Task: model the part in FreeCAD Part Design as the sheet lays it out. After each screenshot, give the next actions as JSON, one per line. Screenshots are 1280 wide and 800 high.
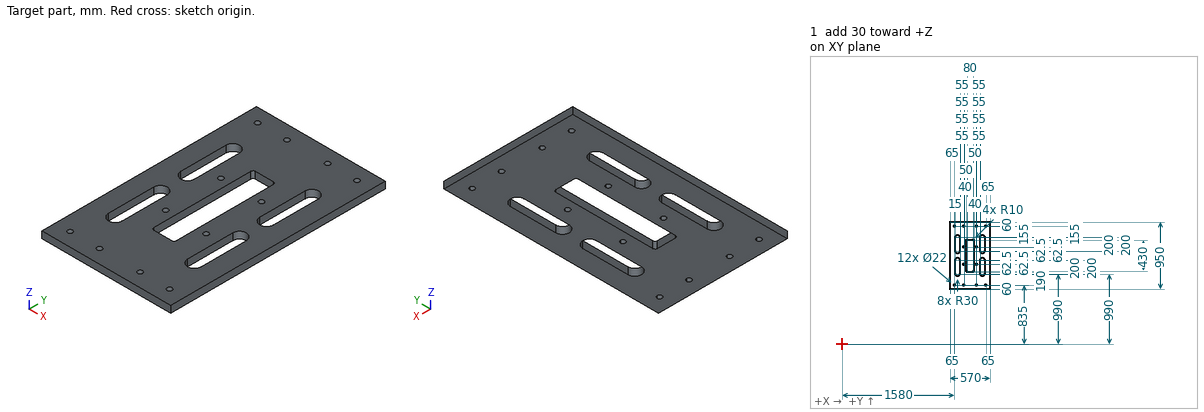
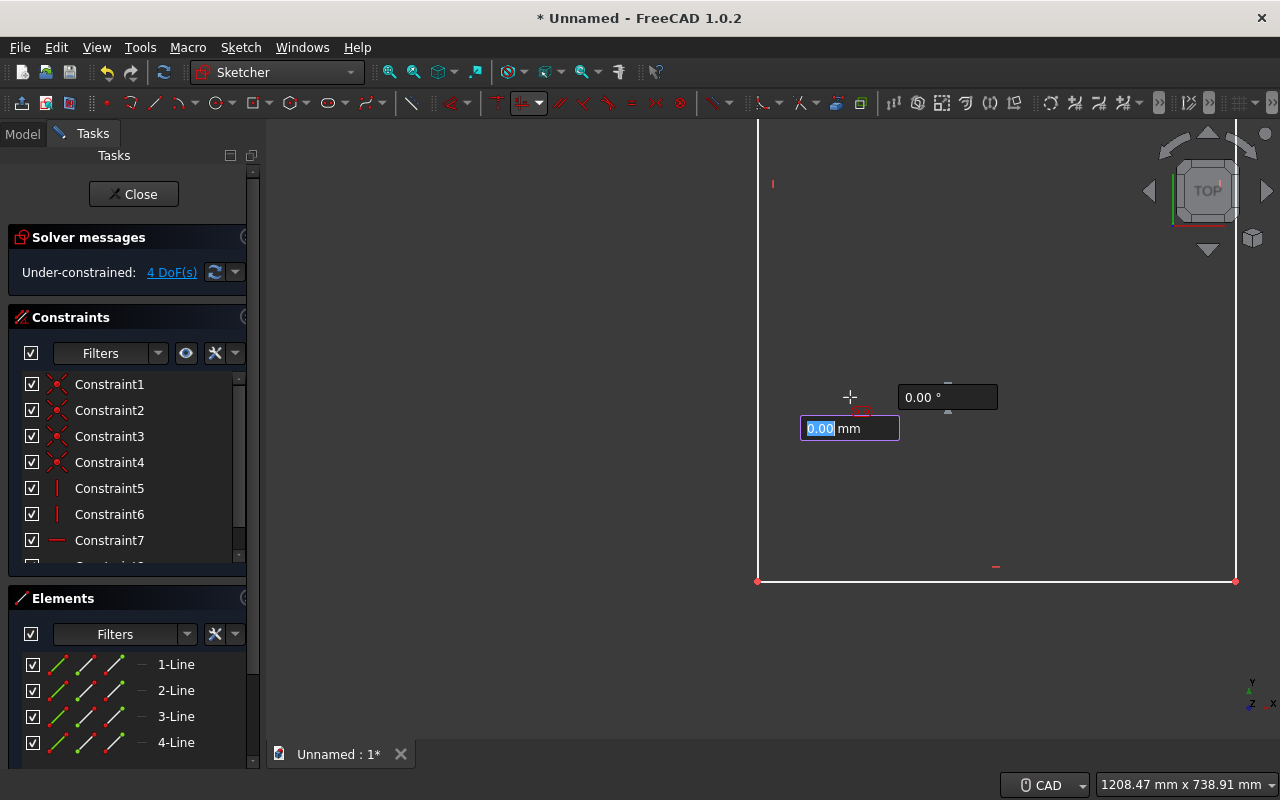
{"action": "left_click", "coordinate": [850, 229]}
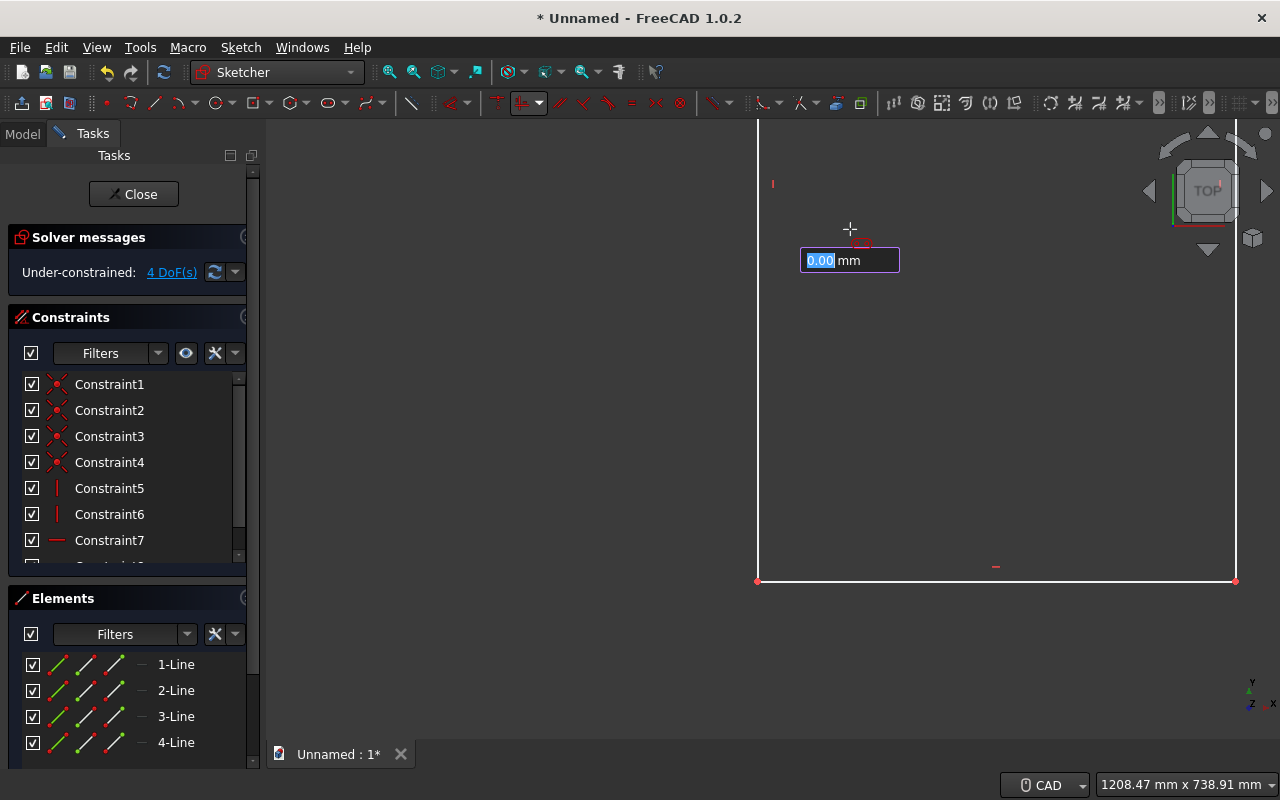
{"action": "left_click", "coordinate": [876, 313]}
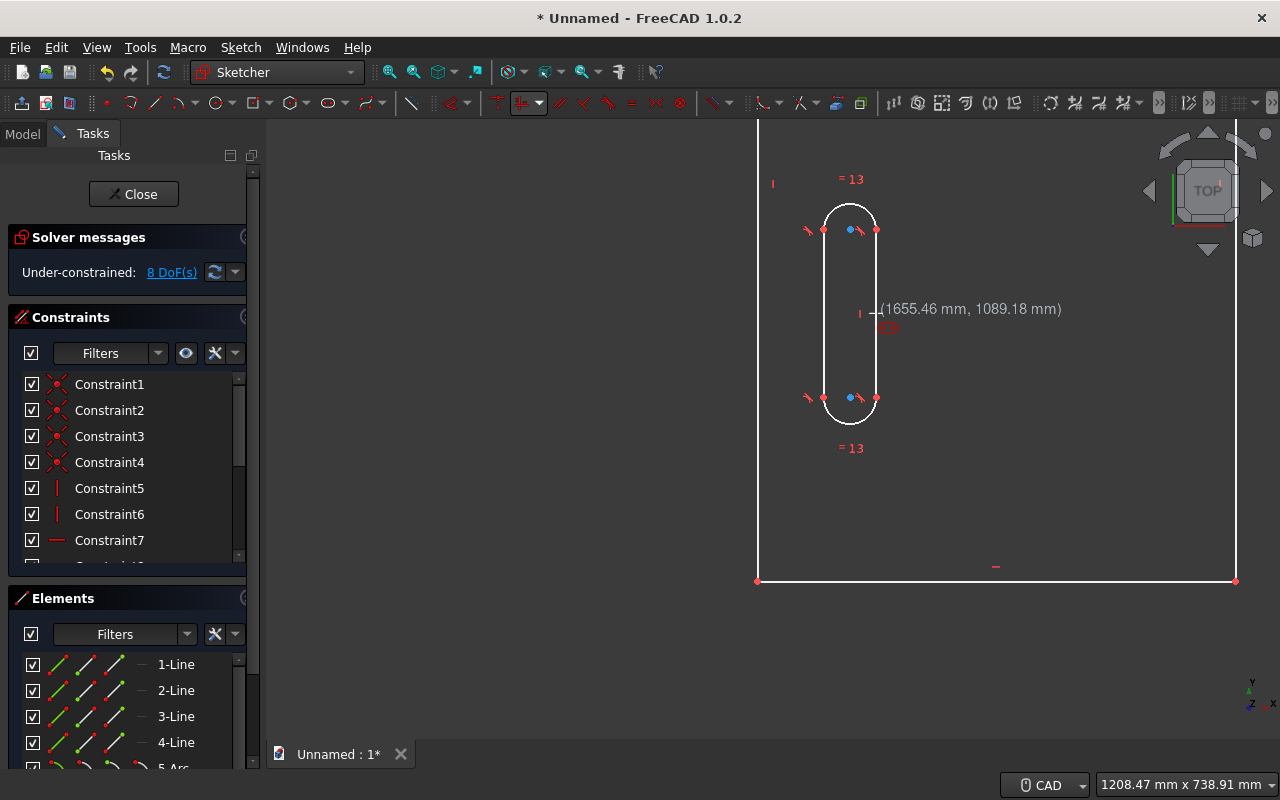
{"action": "scroll", "coordinate": [852, 397], "scroll_direction": "down", "scroll_amount": 6}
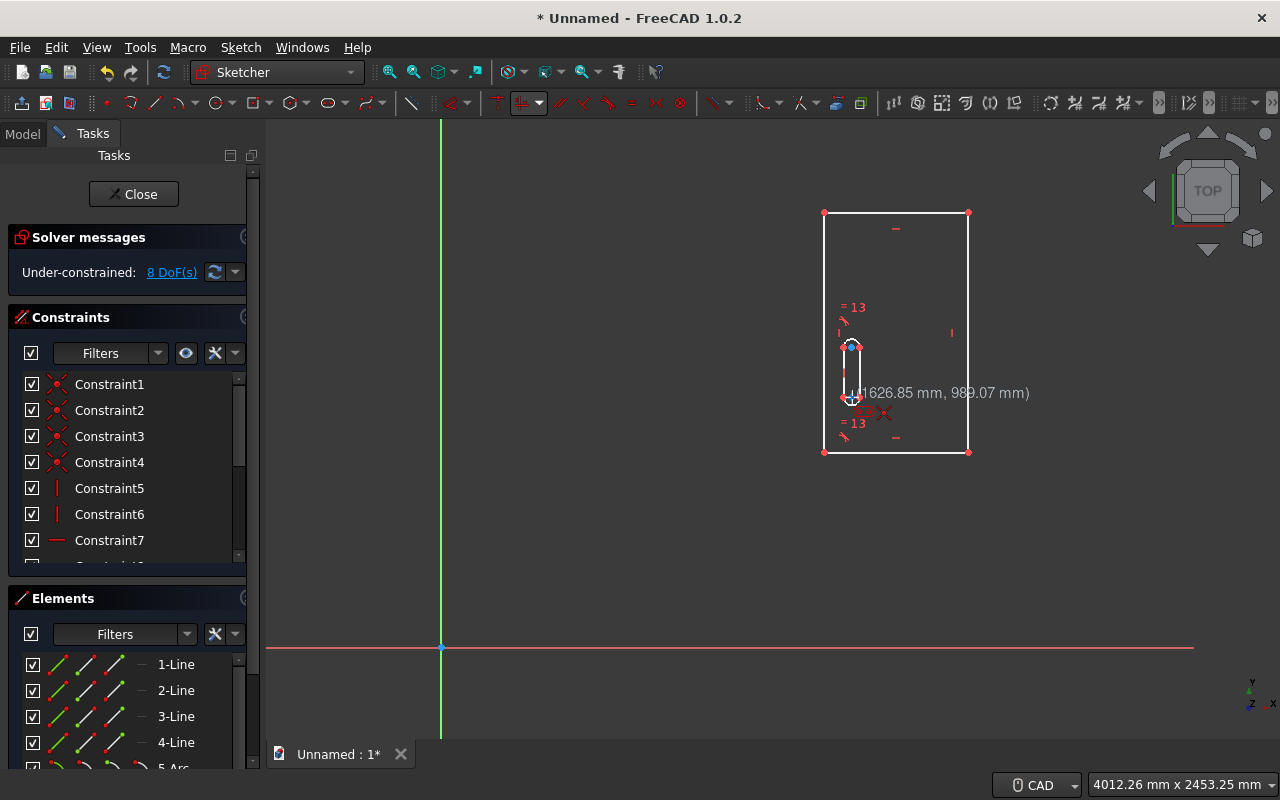
{"action": "scroll", "coordinate": [940, 397], "scroll_direction": "up", "scroll_amount": 6}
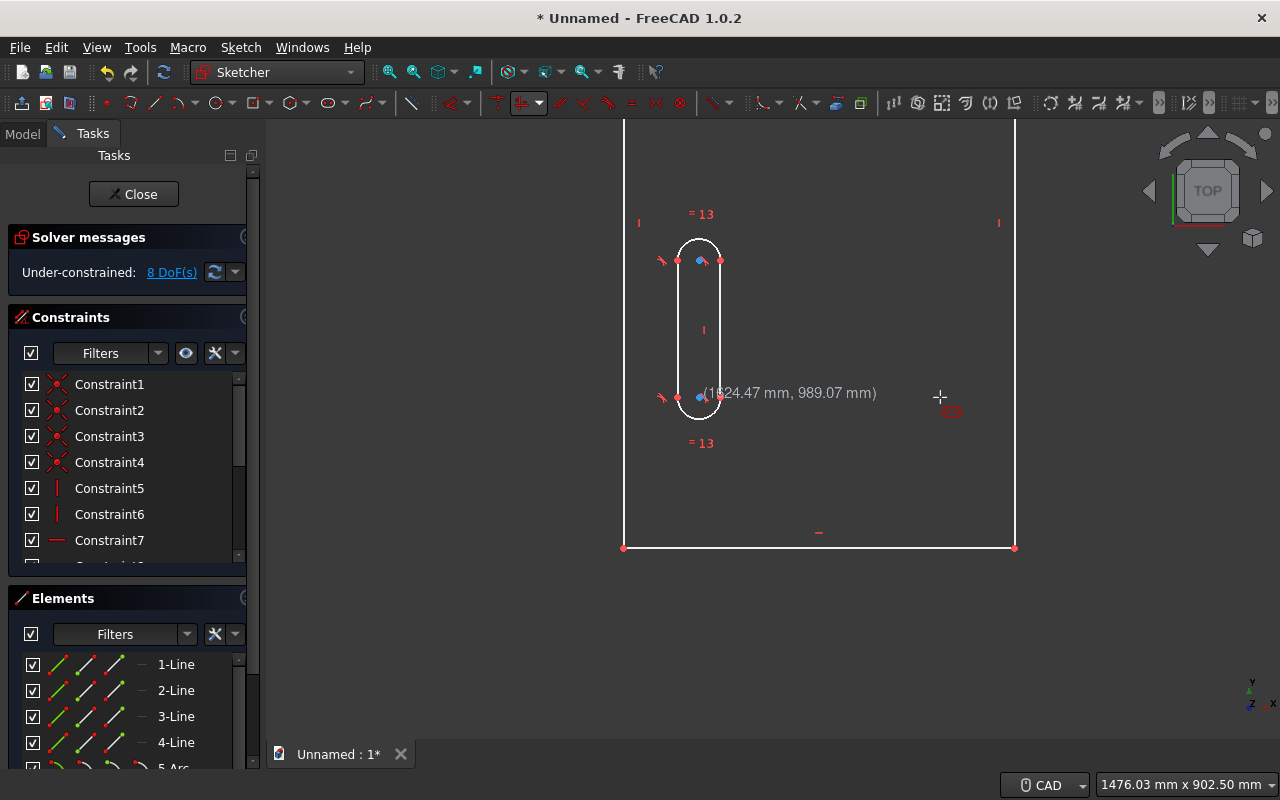
{"action": "left_click", "coordinate": [940, 397]}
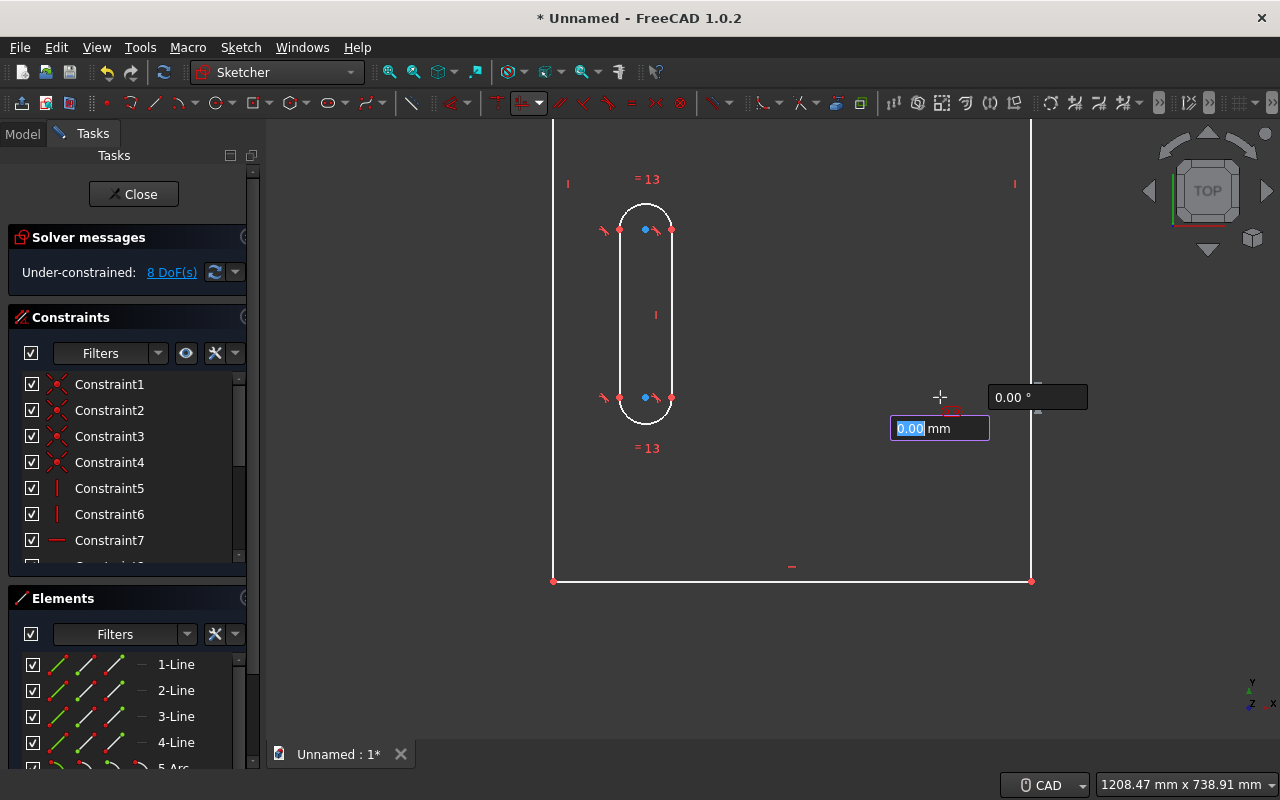
{"action": "left_click", "coordinate": [940, 229]}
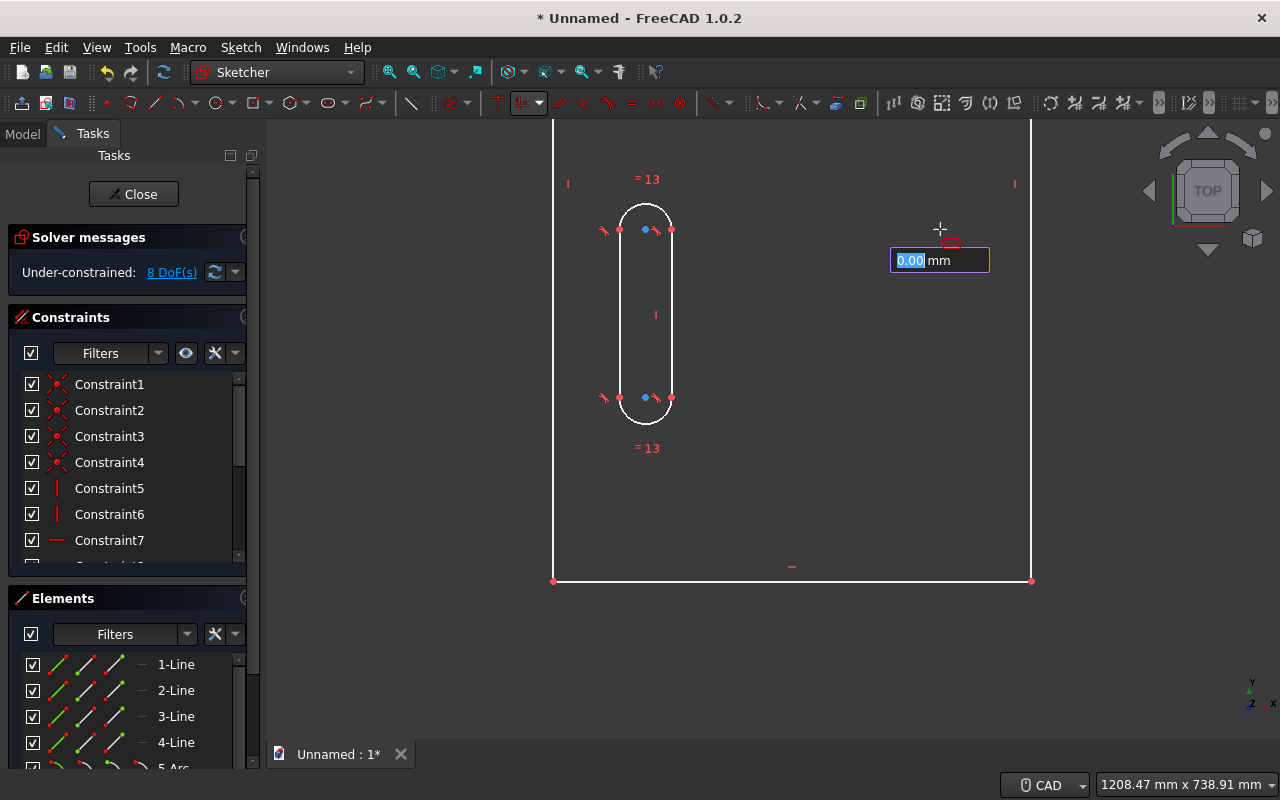
{"action": "left_click", "coordinate": [965, 313]}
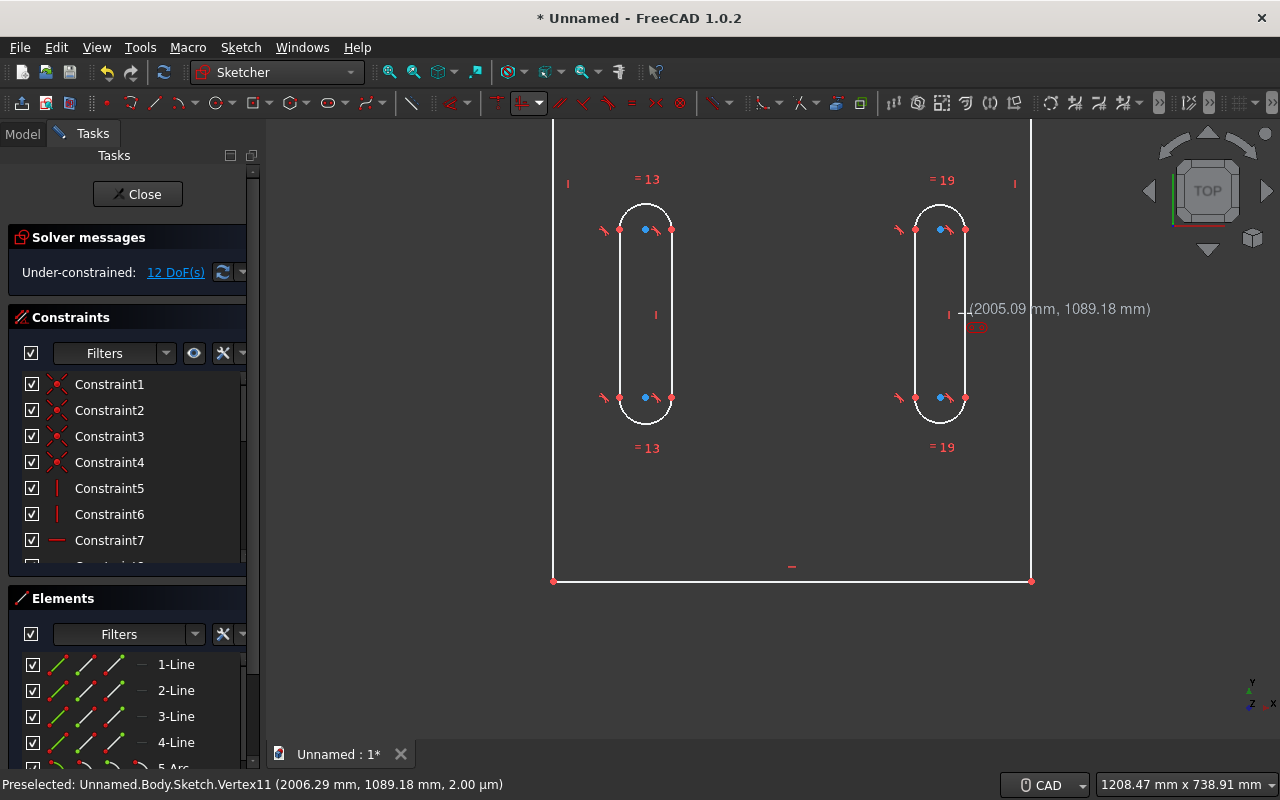
{"action": "scroll", "coordinate": [940, 397], "scroll_direction": "down", "scroll_amount": 6}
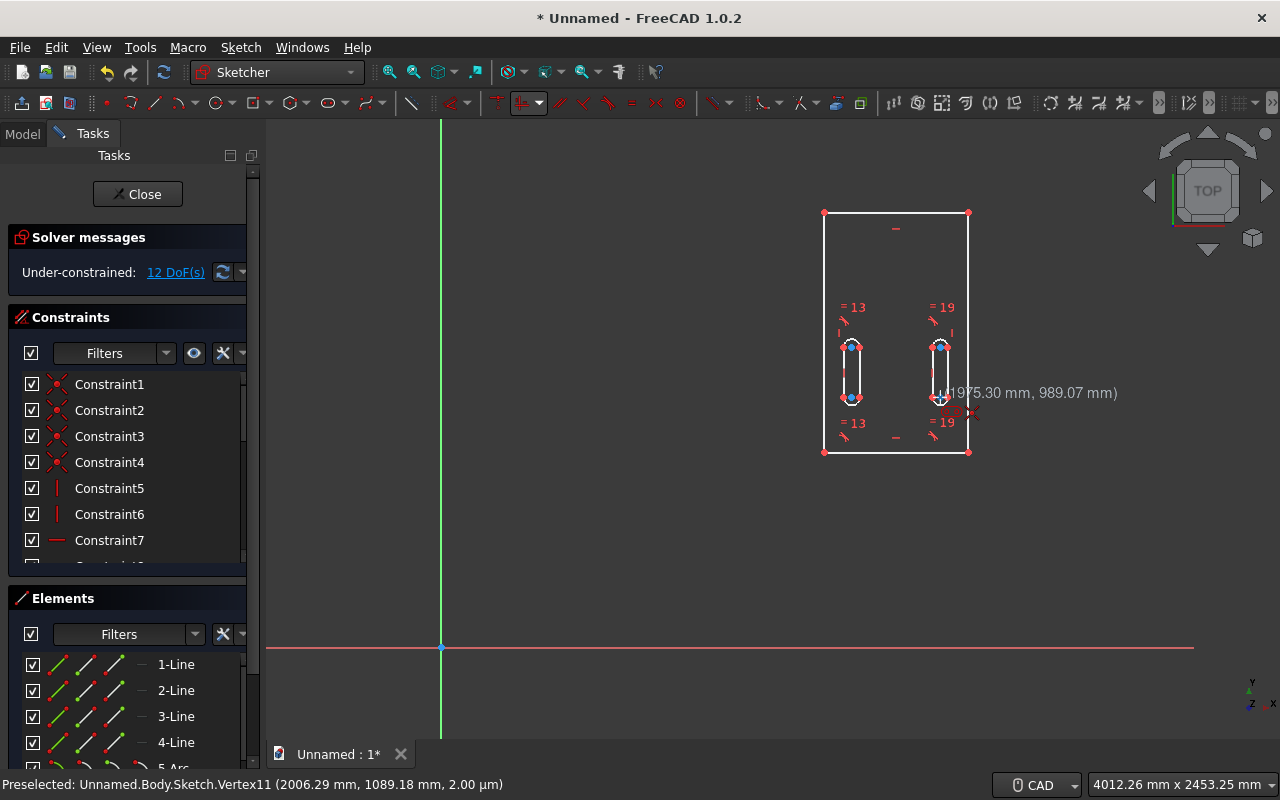
{"action": "scroll", "coordinate": [852, 317], "scroll_direction": "up", "scroll_amount": 6}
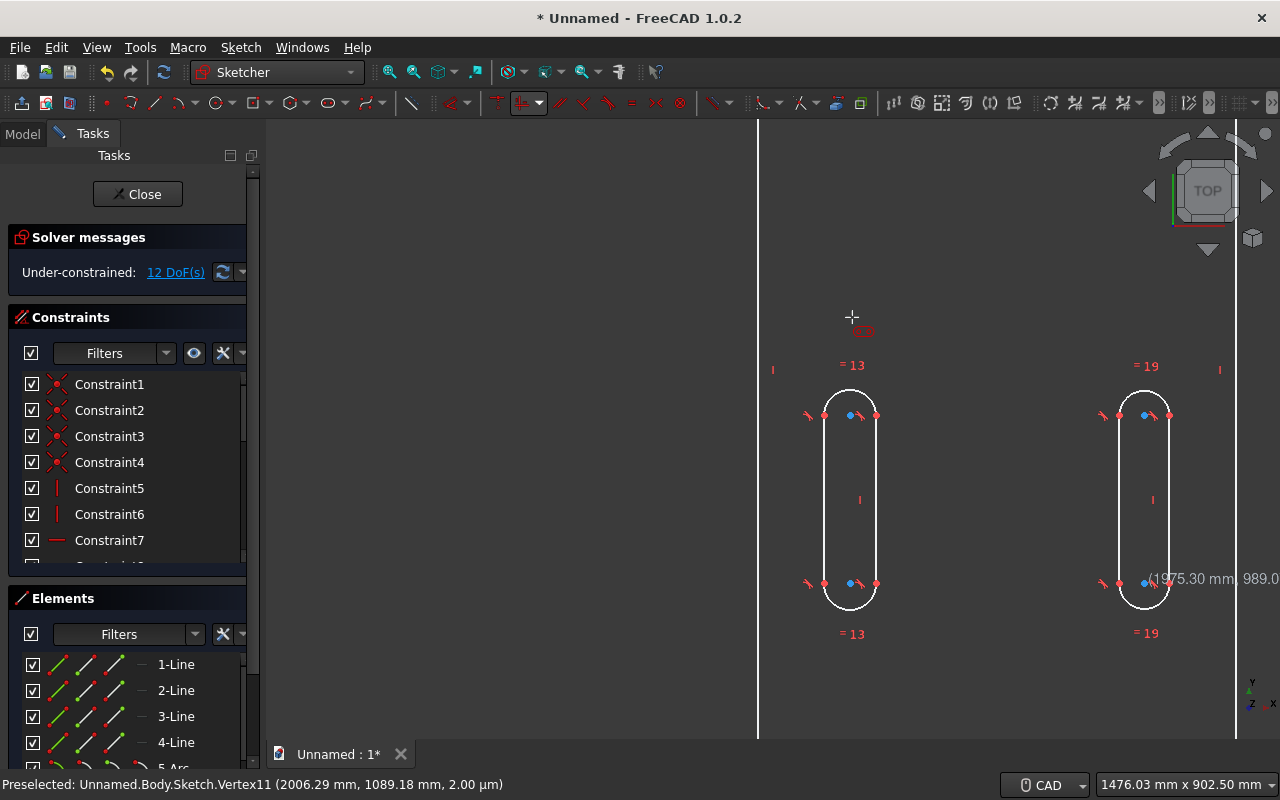
{"action": "left_click", "coordinate": [850, 315]}